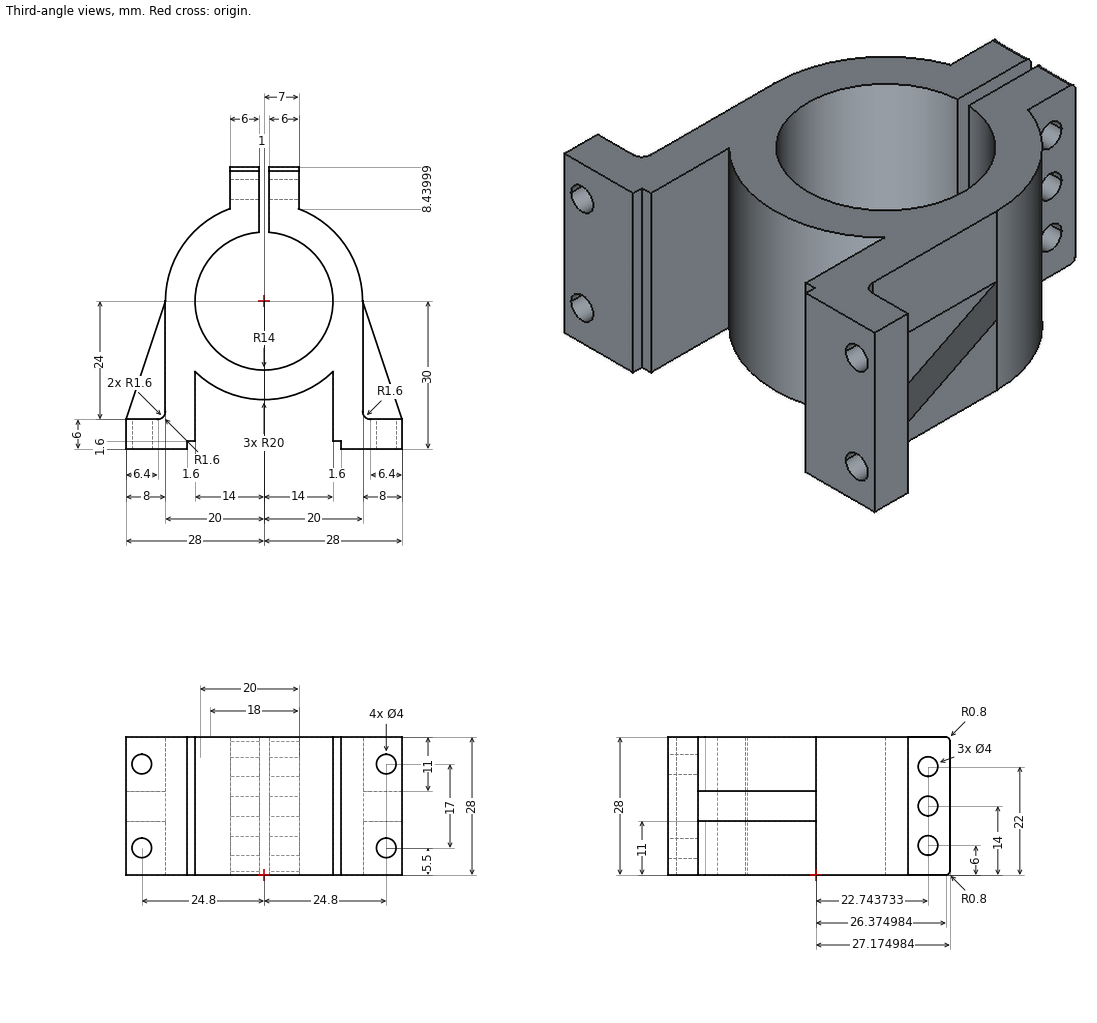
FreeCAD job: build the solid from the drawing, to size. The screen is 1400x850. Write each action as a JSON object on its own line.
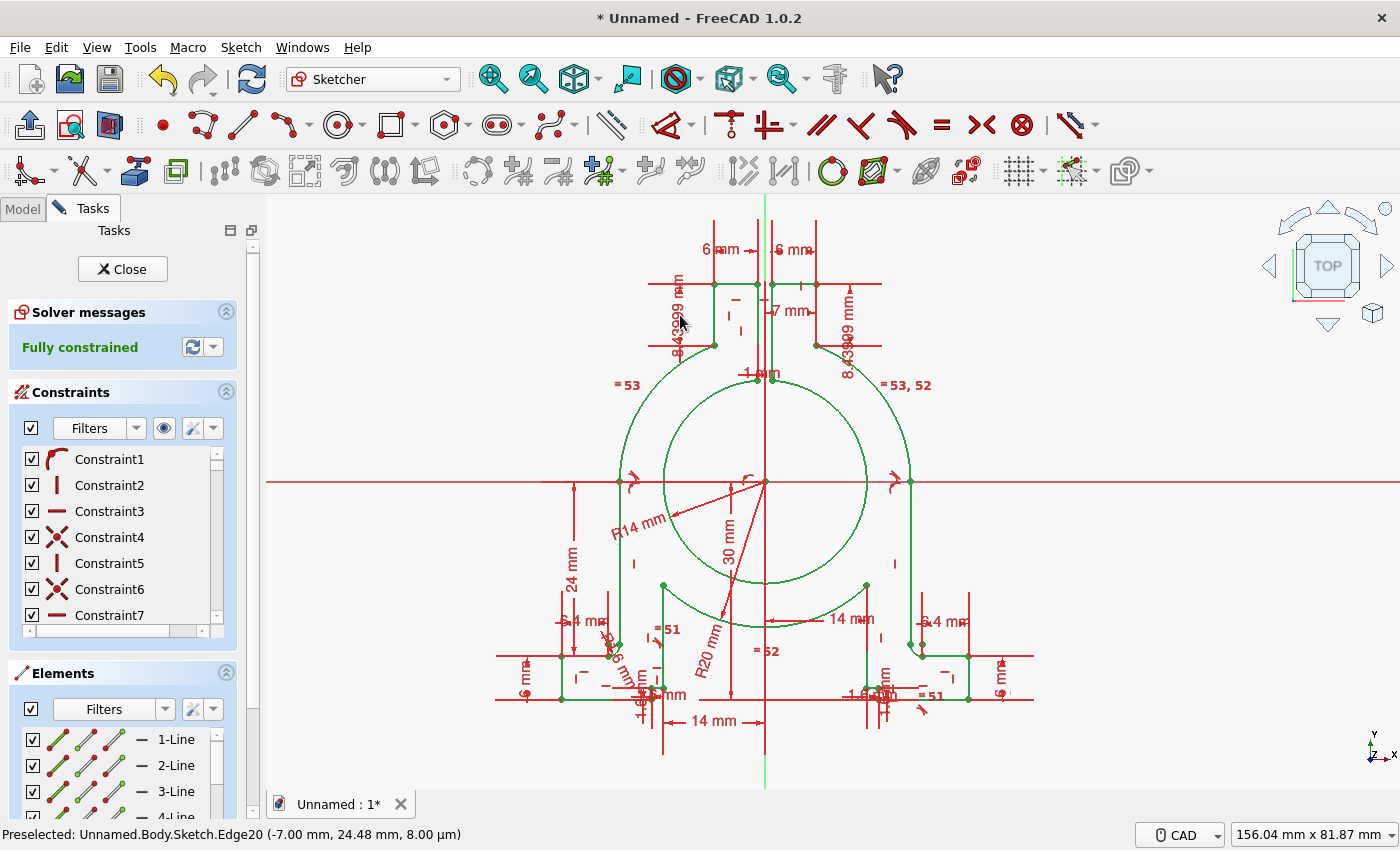
{"action": "left_click", "coordinate": [123, 269]}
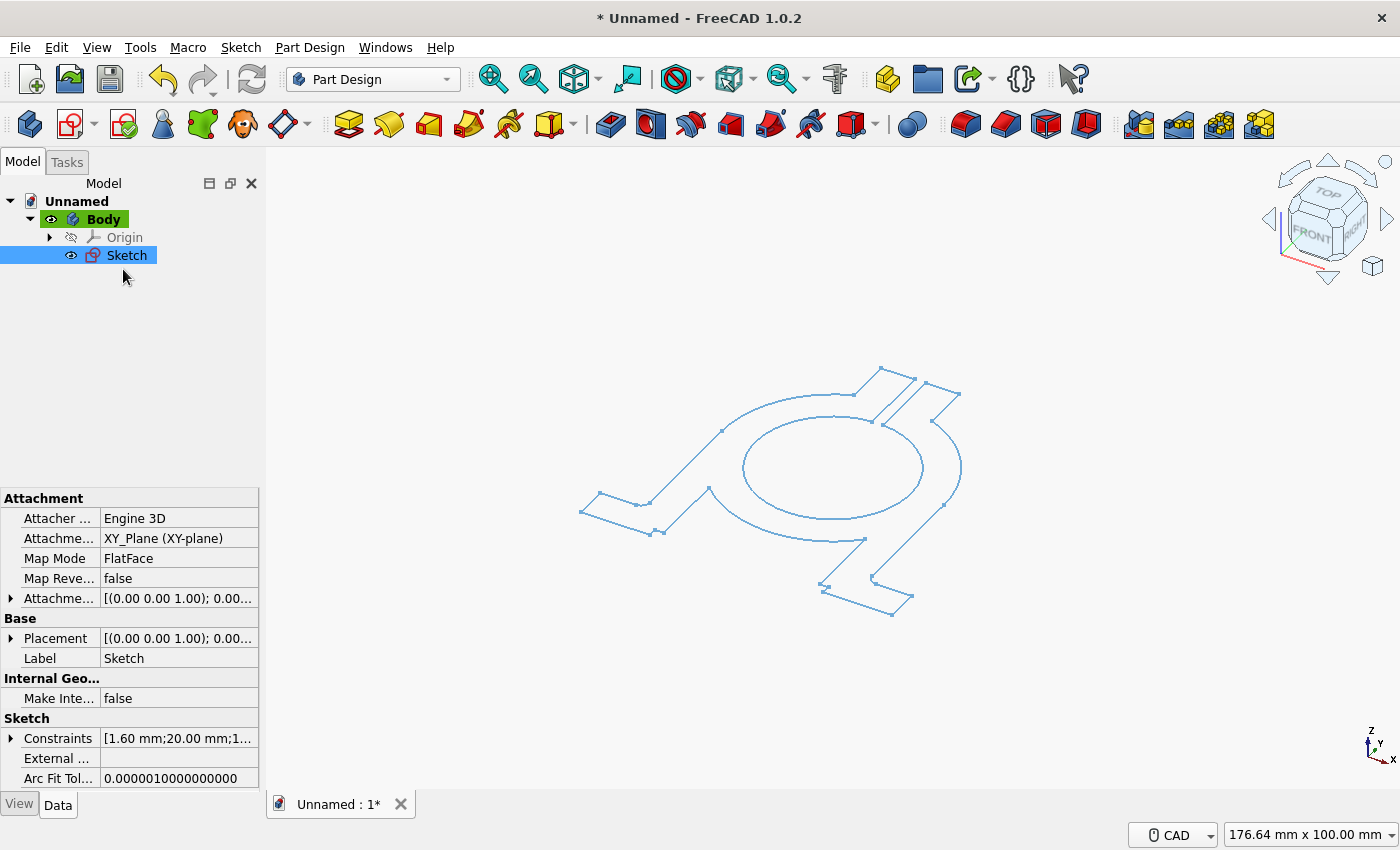
{"action": "left_click", "coordinate": [350, 124]}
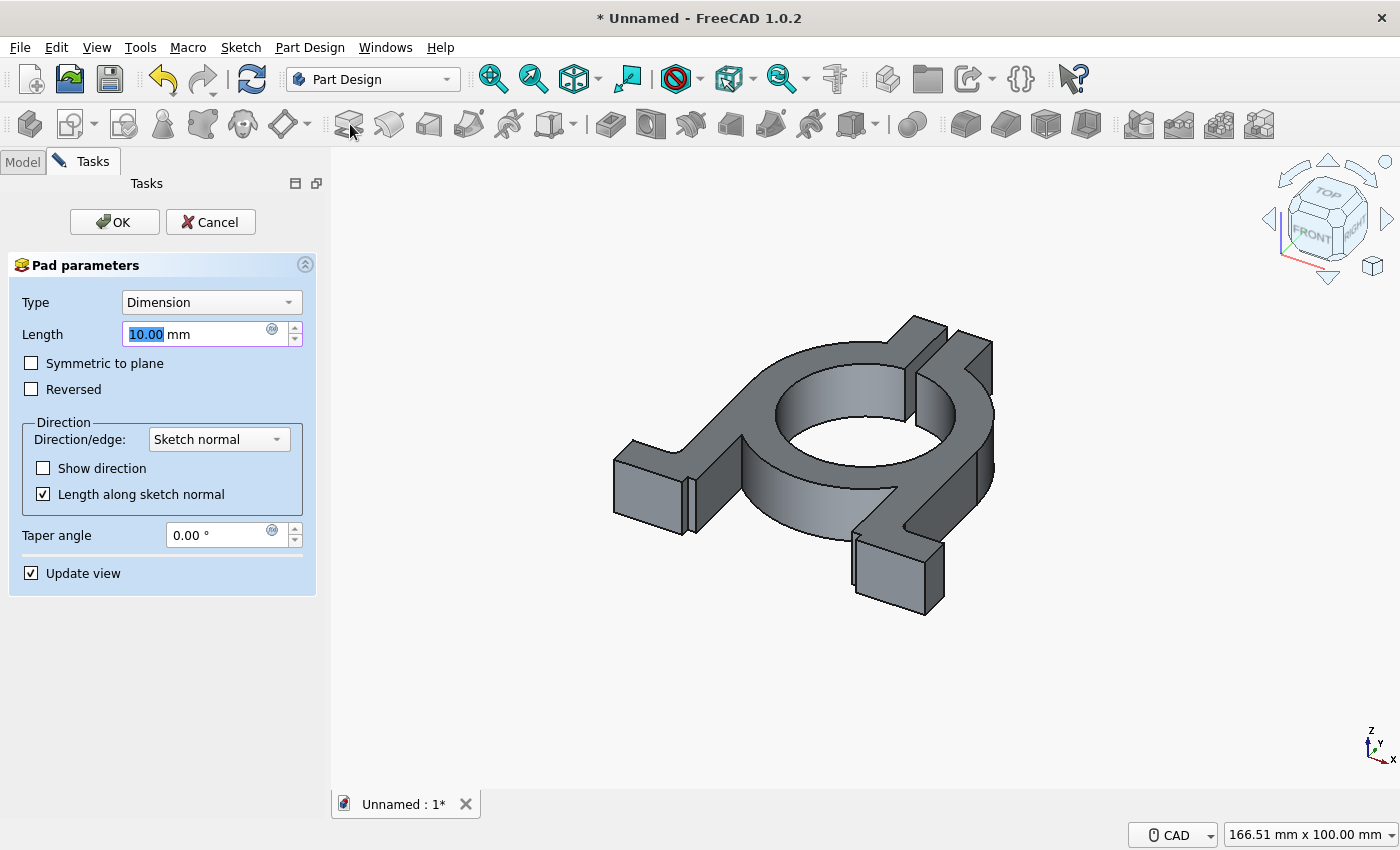
{"action": "type", "text": "28"}
{"action": "key", "text": "Tab"}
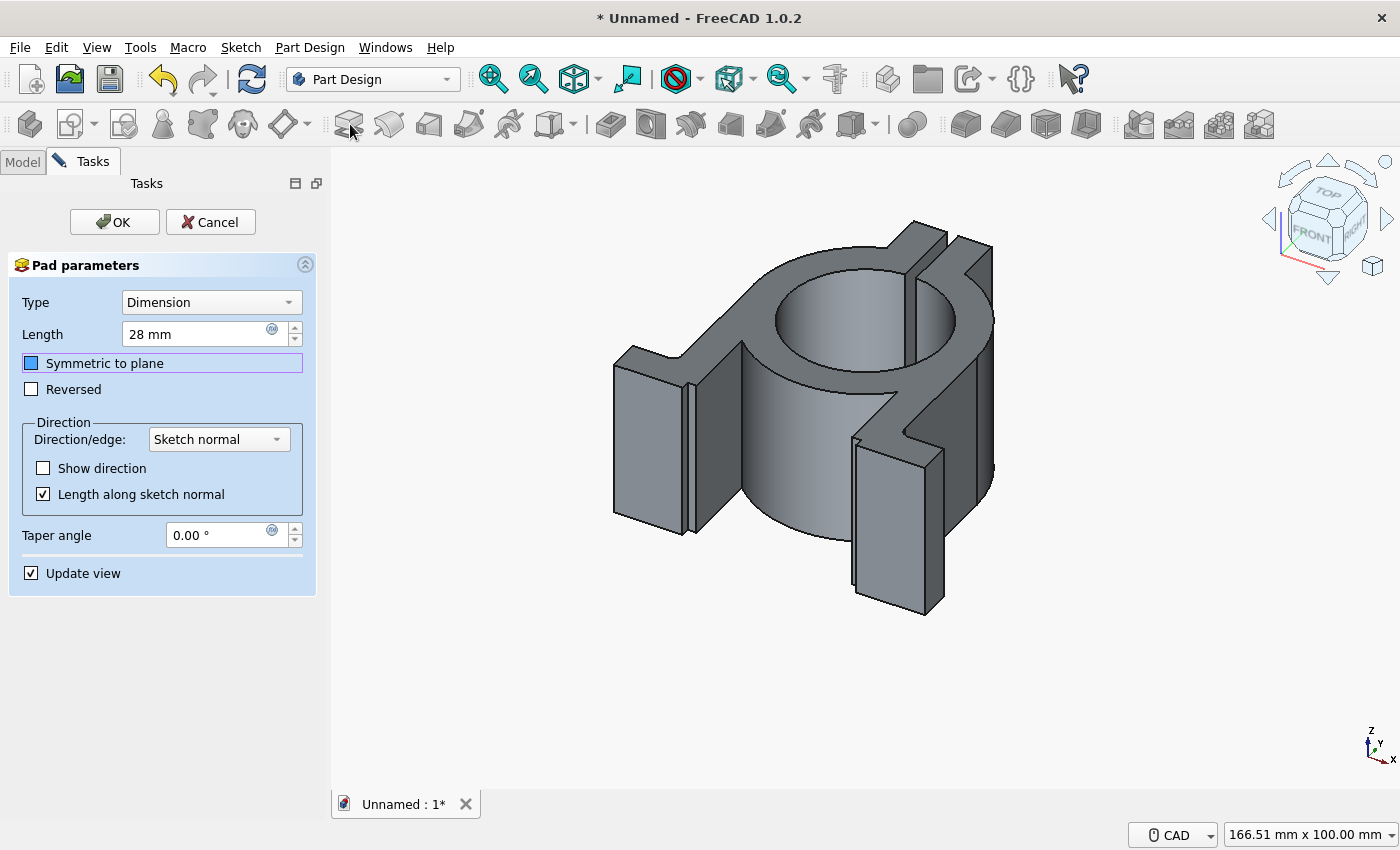
{"action": "left_click", "coordinate": [115, 222]}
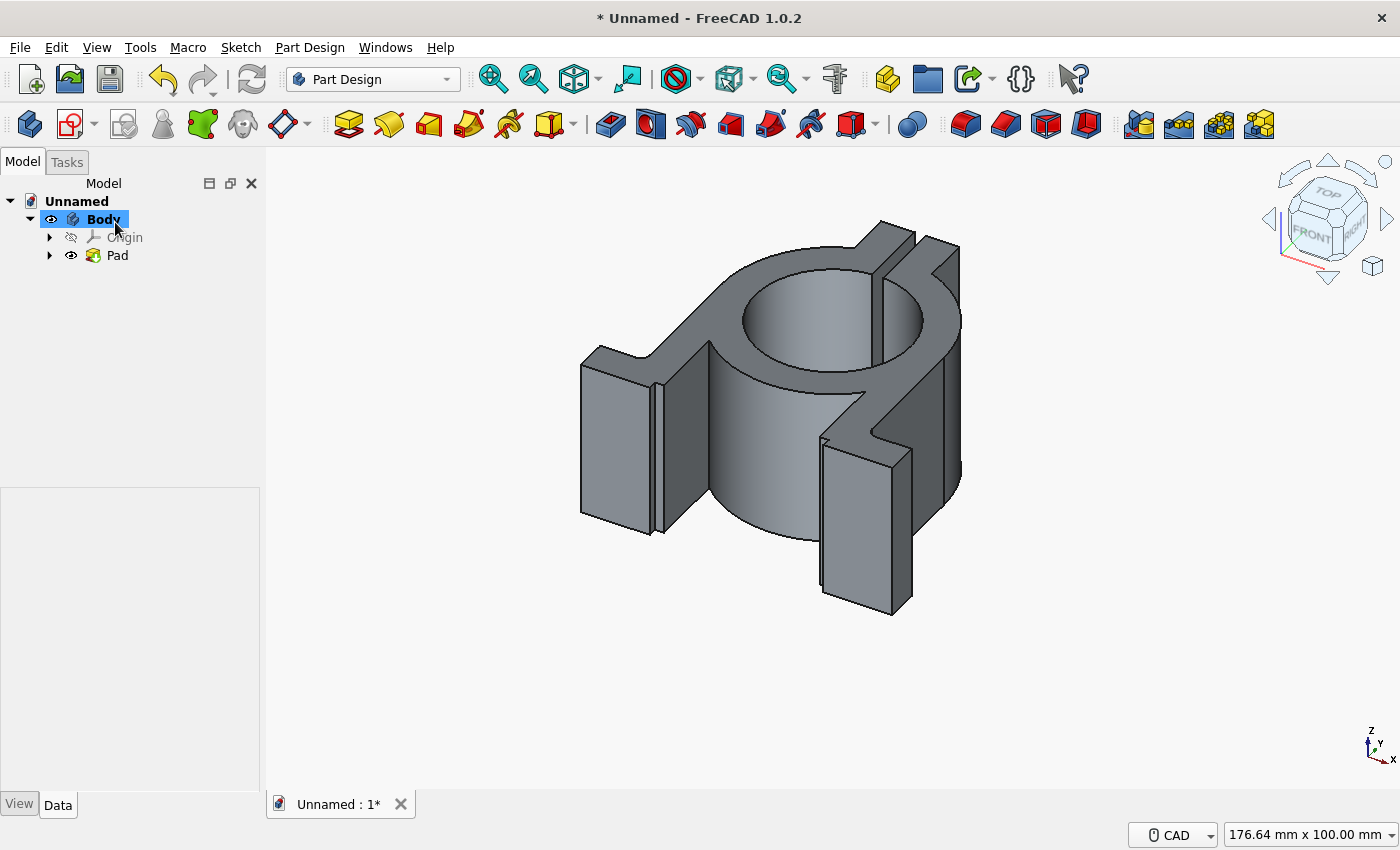
{"action": "key", "text": "0"}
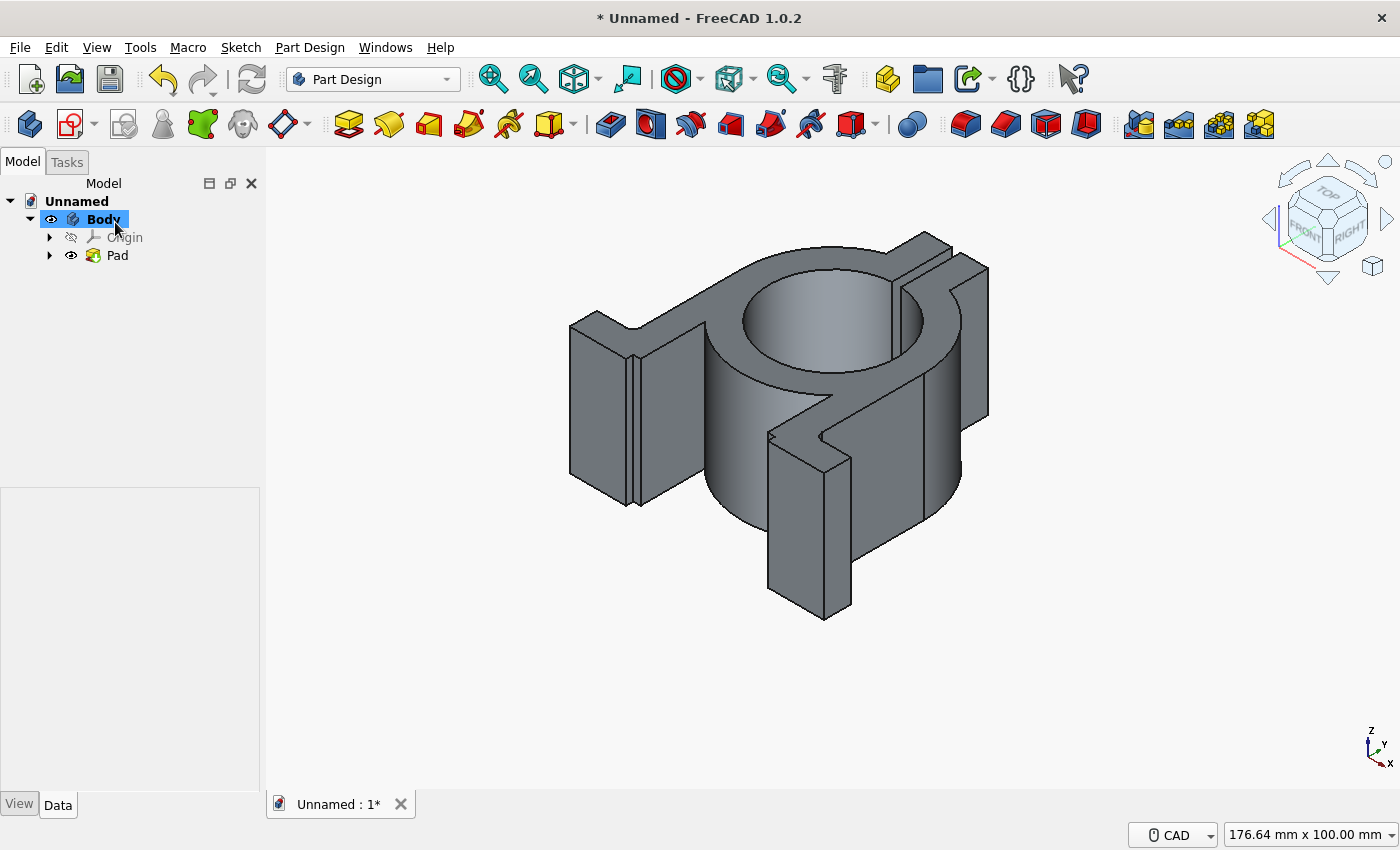
{"action": "left_click", "coordinate": [969, 310]}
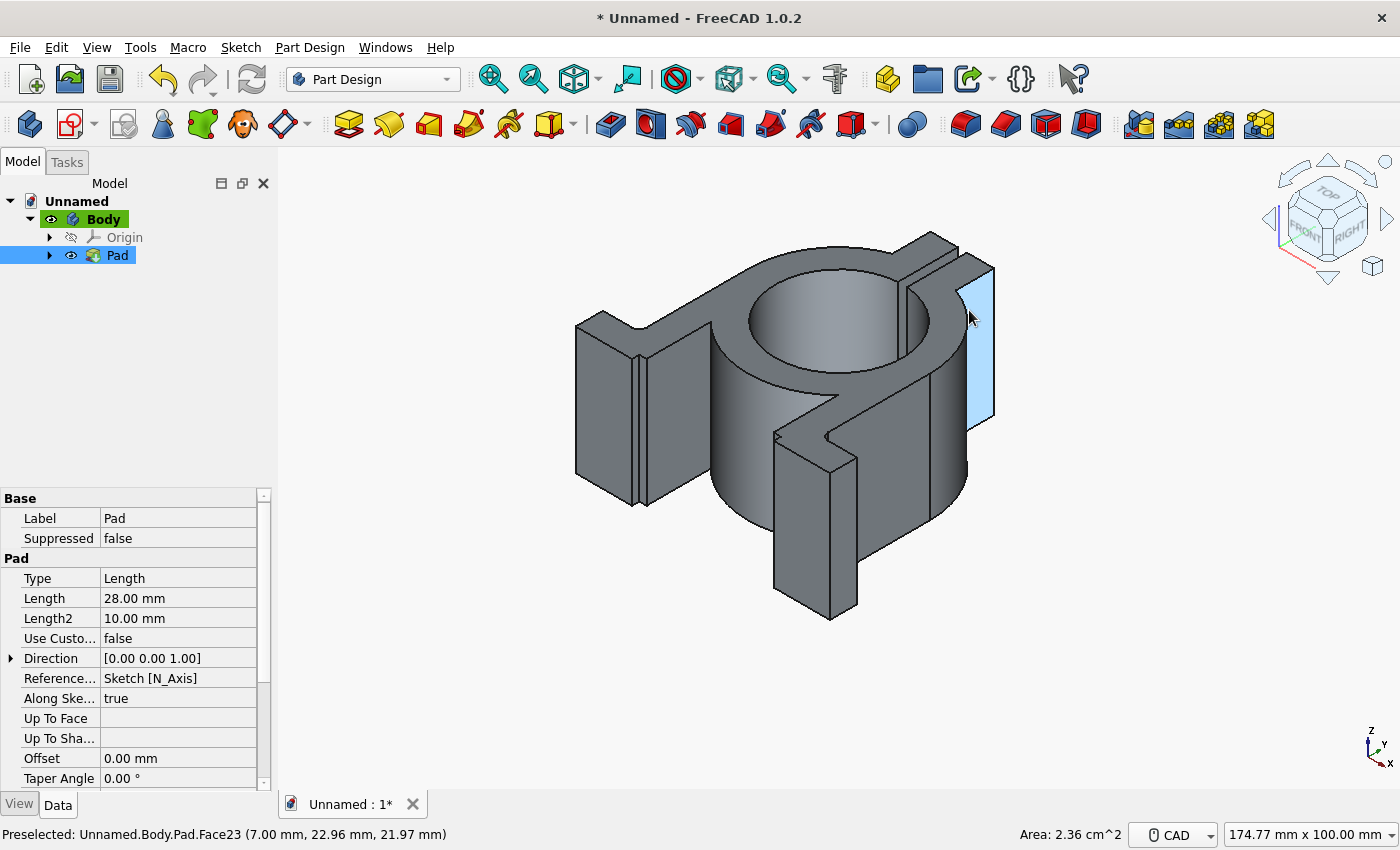
{"action": "left_click", "coordinate": [70, 124]}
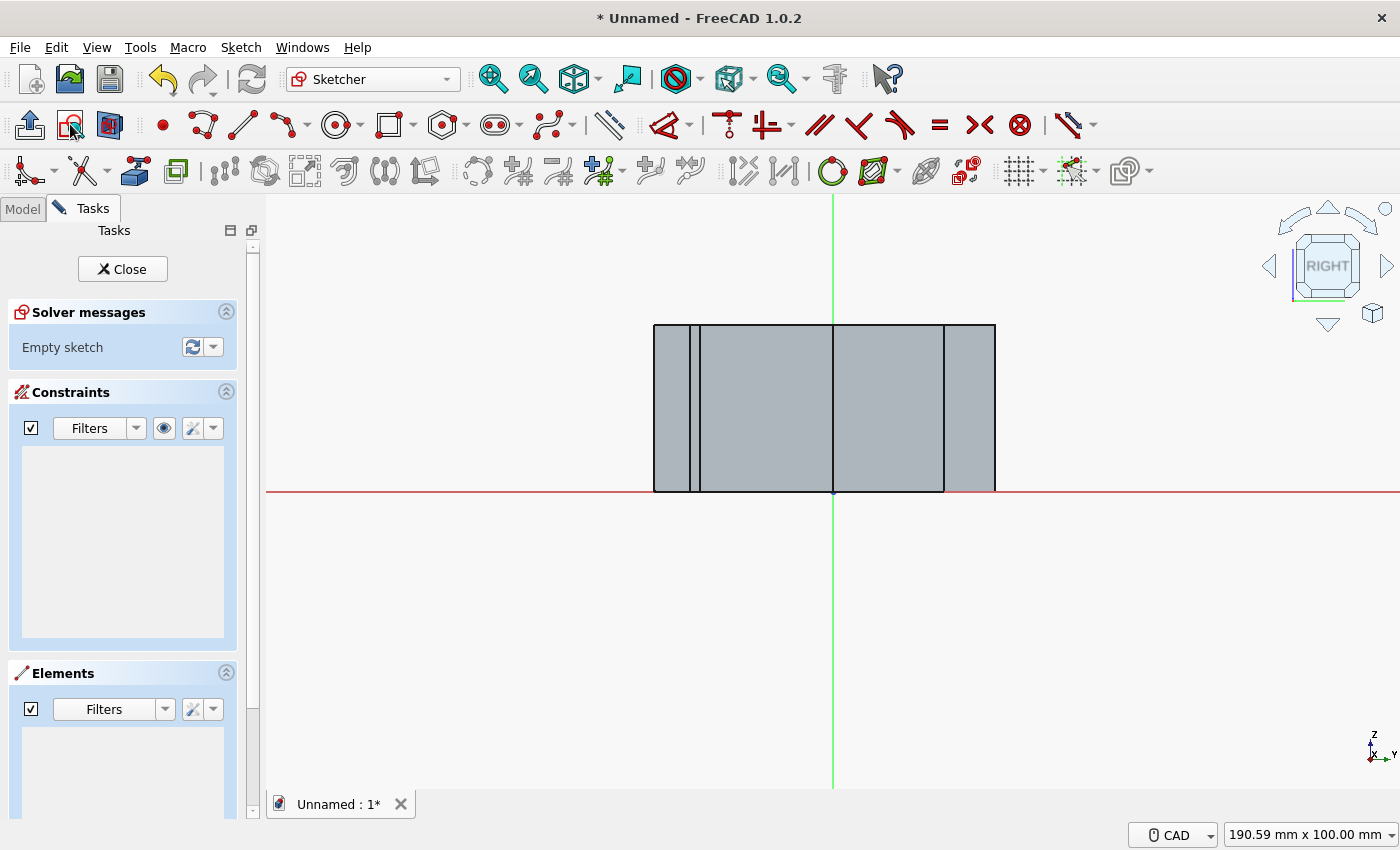
{"action": "scroll", "coordinate": [1004, 319], "scroll_direction": "up", "scroll_amount": 15}